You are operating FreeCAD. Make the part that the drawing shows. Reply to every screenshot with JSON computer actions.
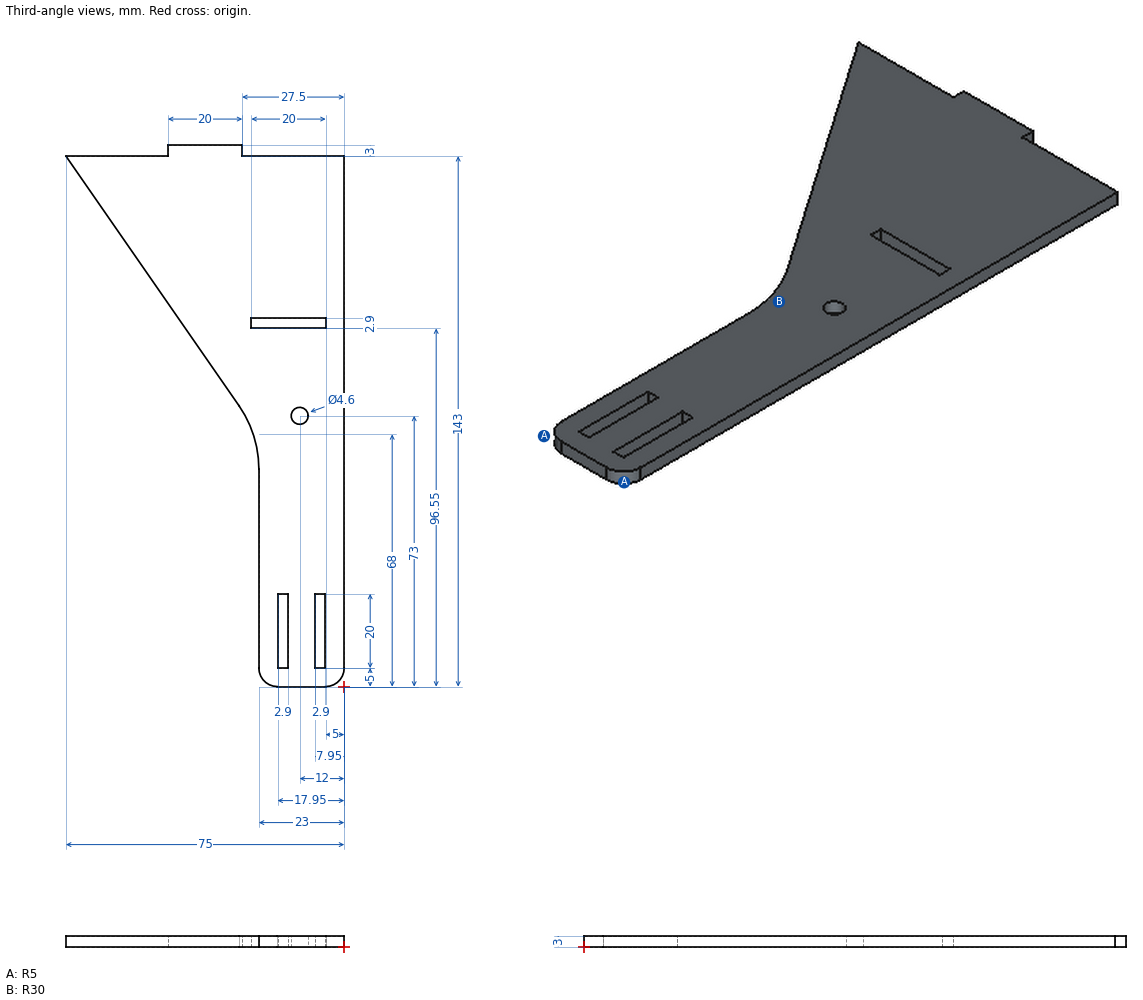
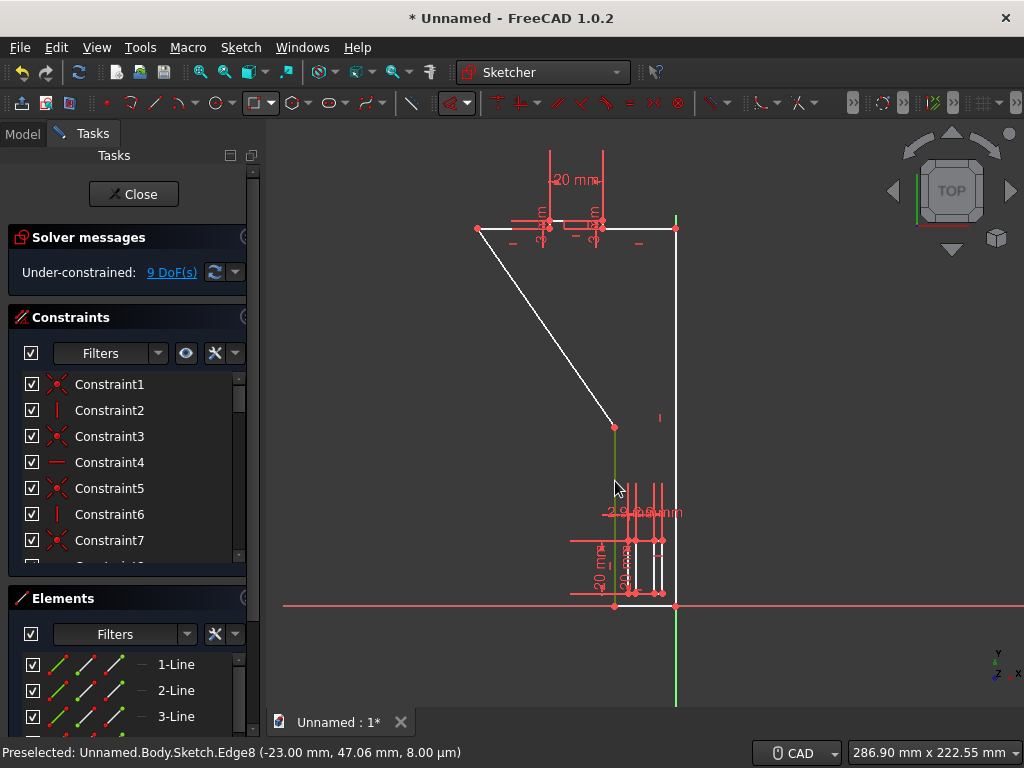
{"action": "left_click", "coordinate": [470, 104]}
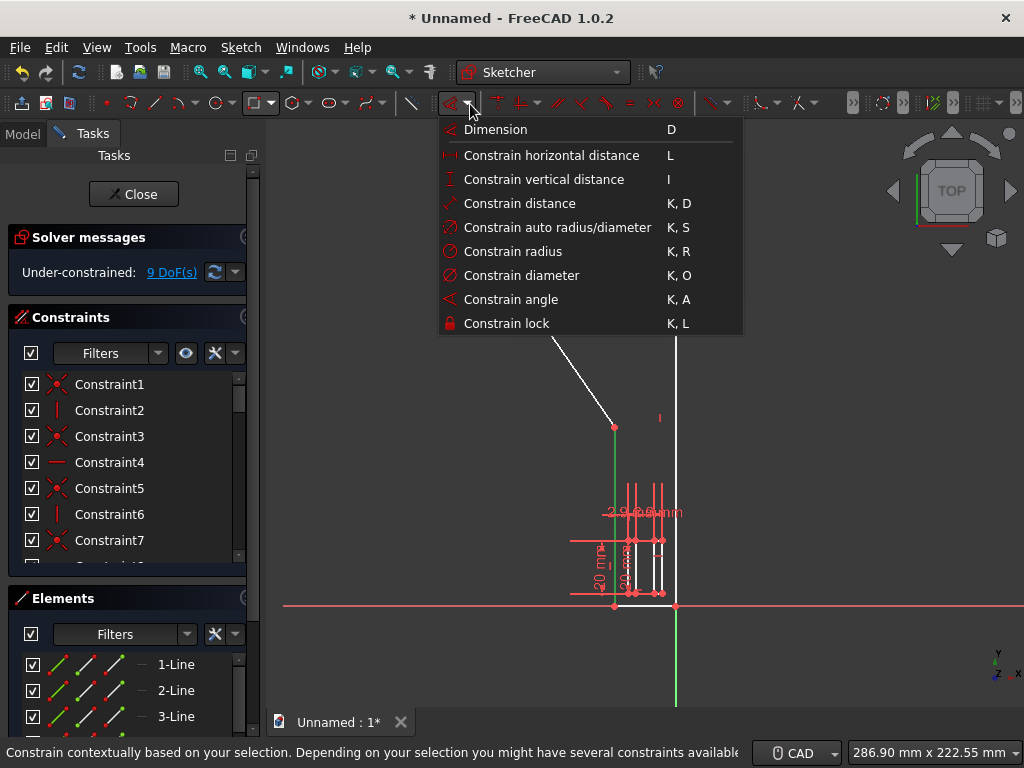
{"action": "left_click", "coordinate": [591, 179]}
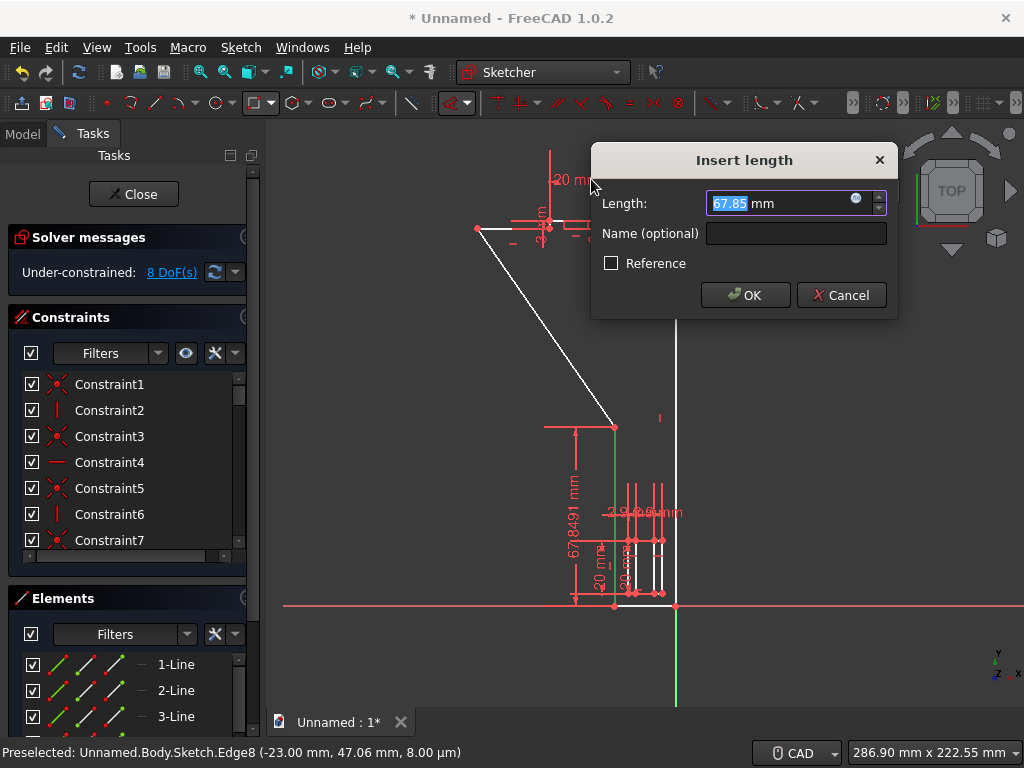
{"action": "type", "text": "68"}
{"action": "key", "text": "Return"}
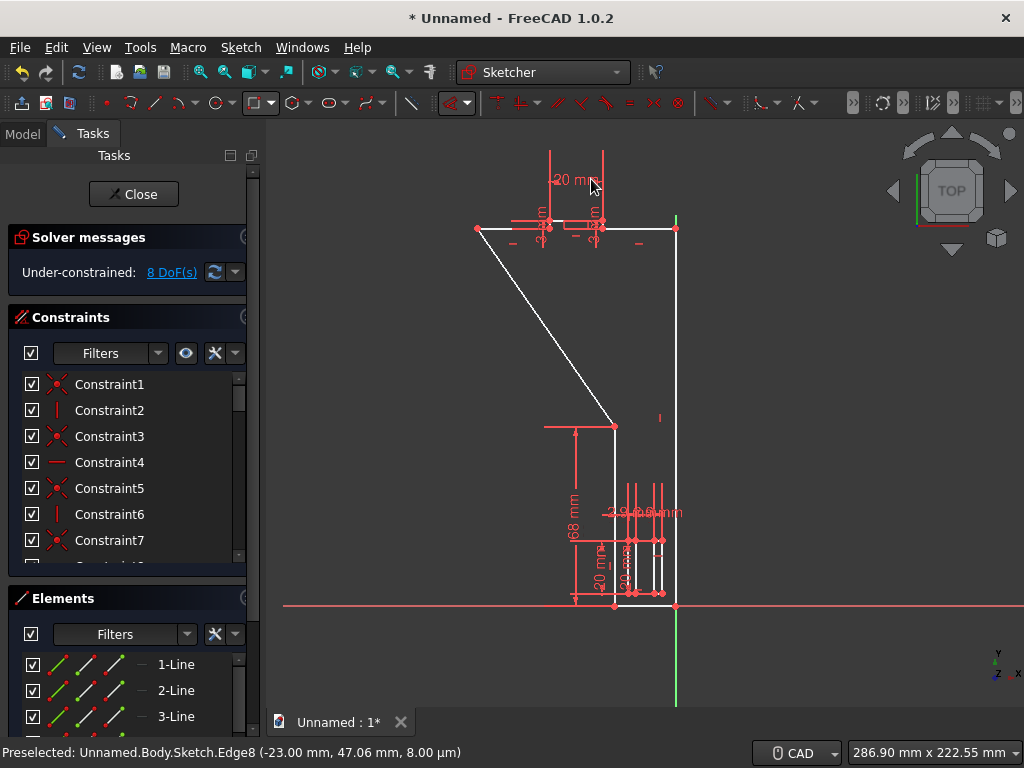
{"action": "left_click", "coordinate": [633, 606]}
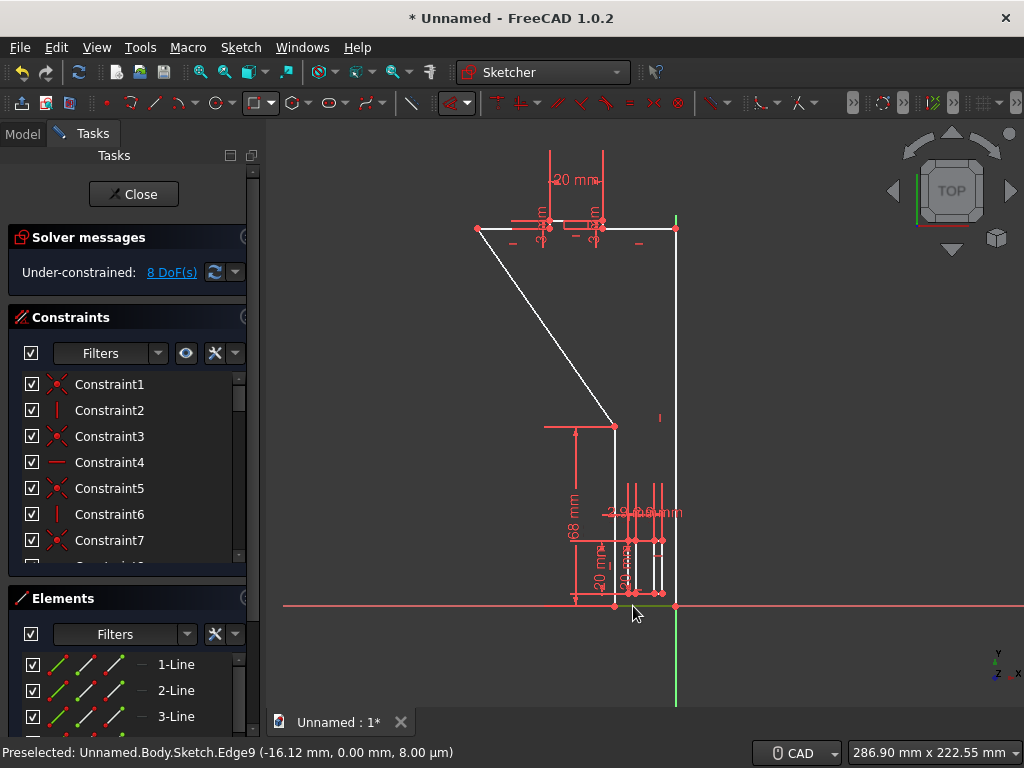
{"action": "key", "text": "l"}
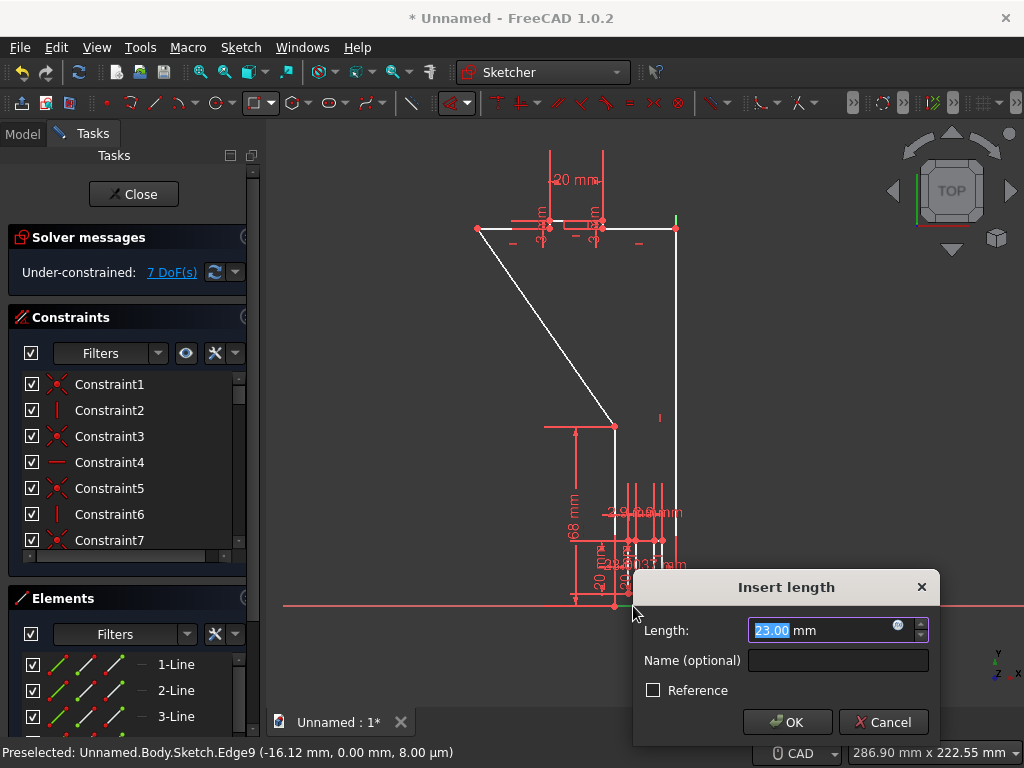
{"action": "type", "text": "23"}
{"action": "key", "text": "Return"}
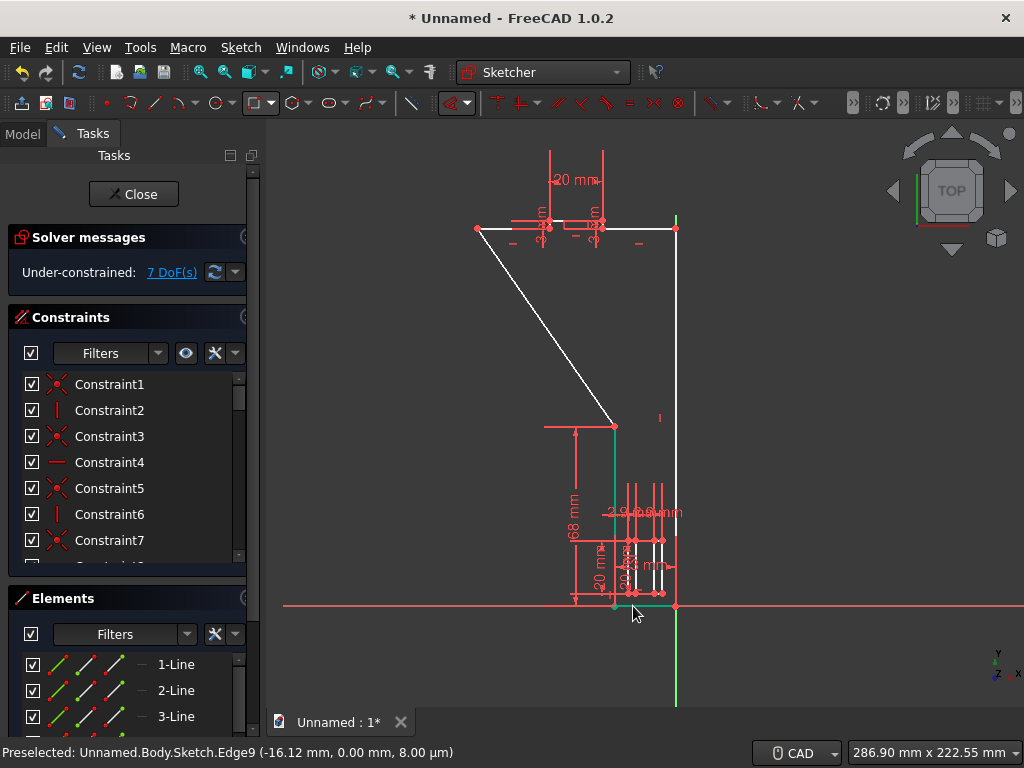
{"action": "scroll", "coordinate": [654, 594], "scroll_direction": "up", "scroll_amount": 6}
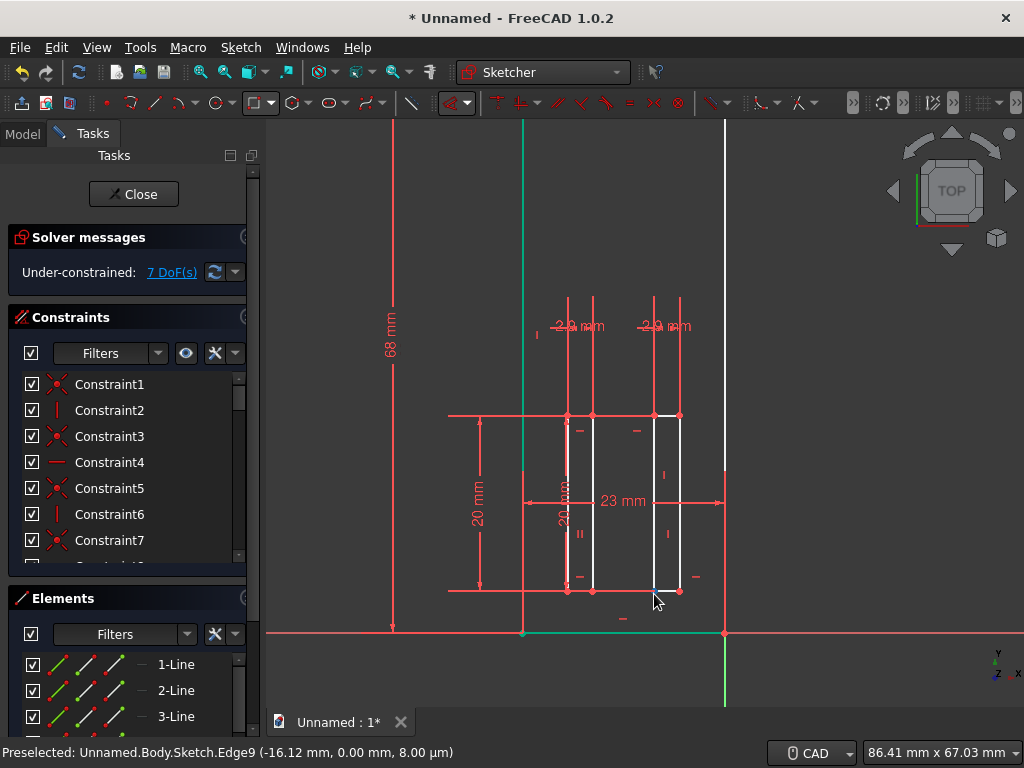
{"action": "left_click", "coordinate": [654, 591]}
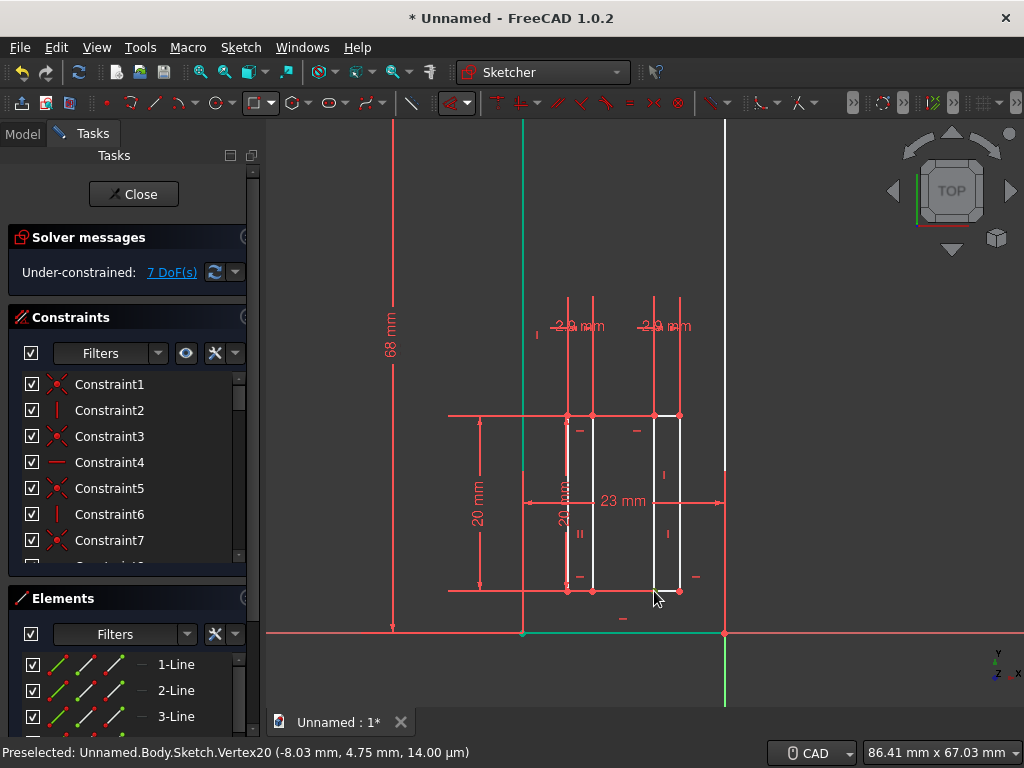
{"action": "key", "text": "i"}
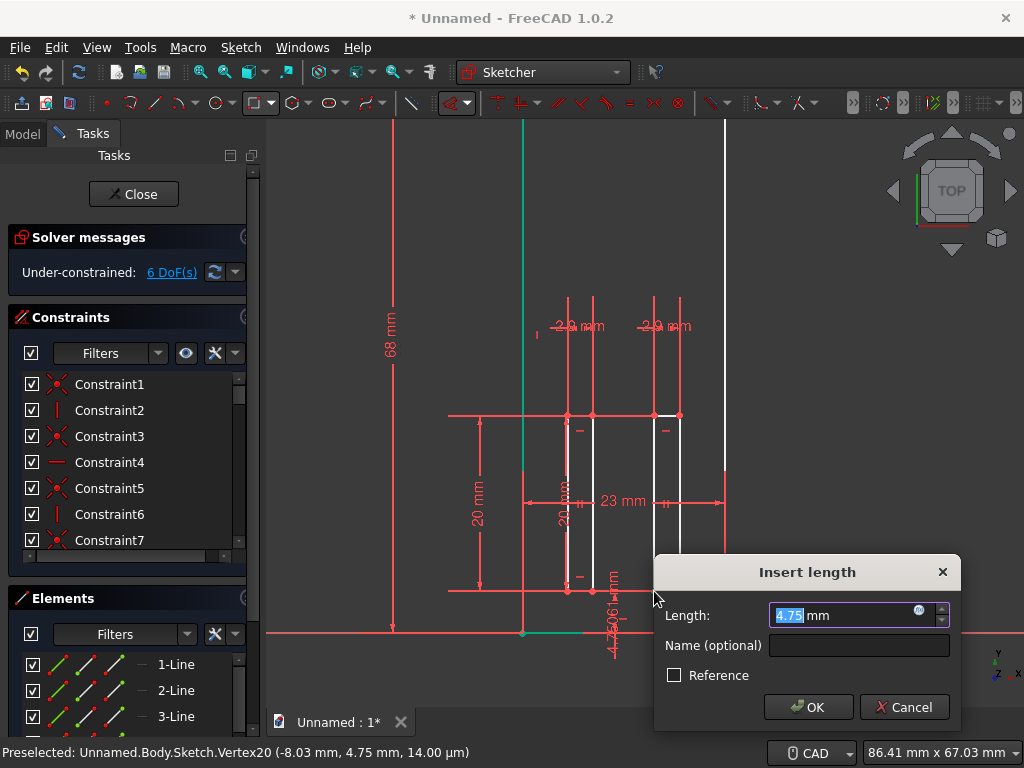
{"action": "type", "text": "5"}
{"action": "key", "text": "Return"}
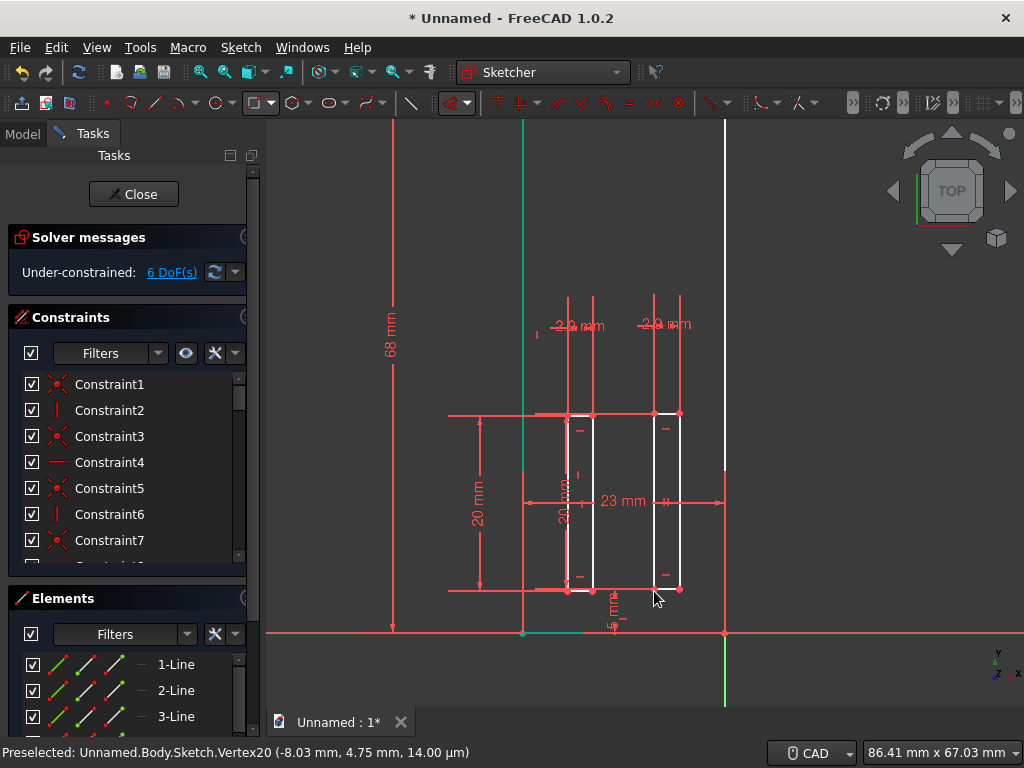
{"action": "left_click", "coordinate": [568, 591]}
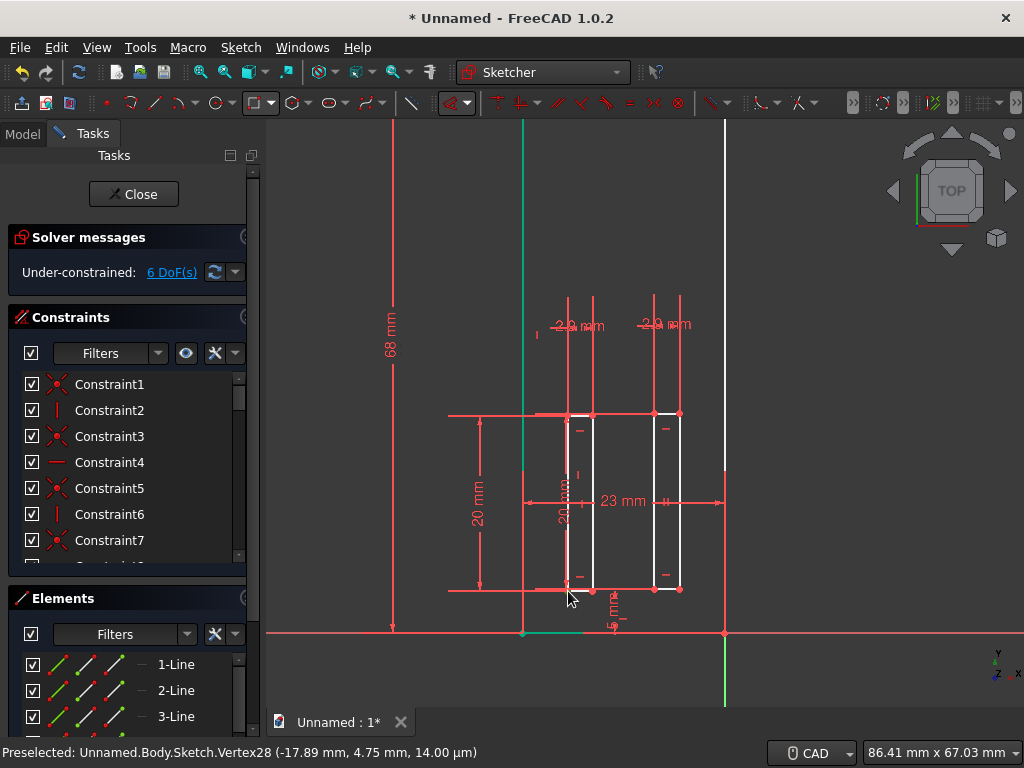
{"action": "key", "text": "i"}